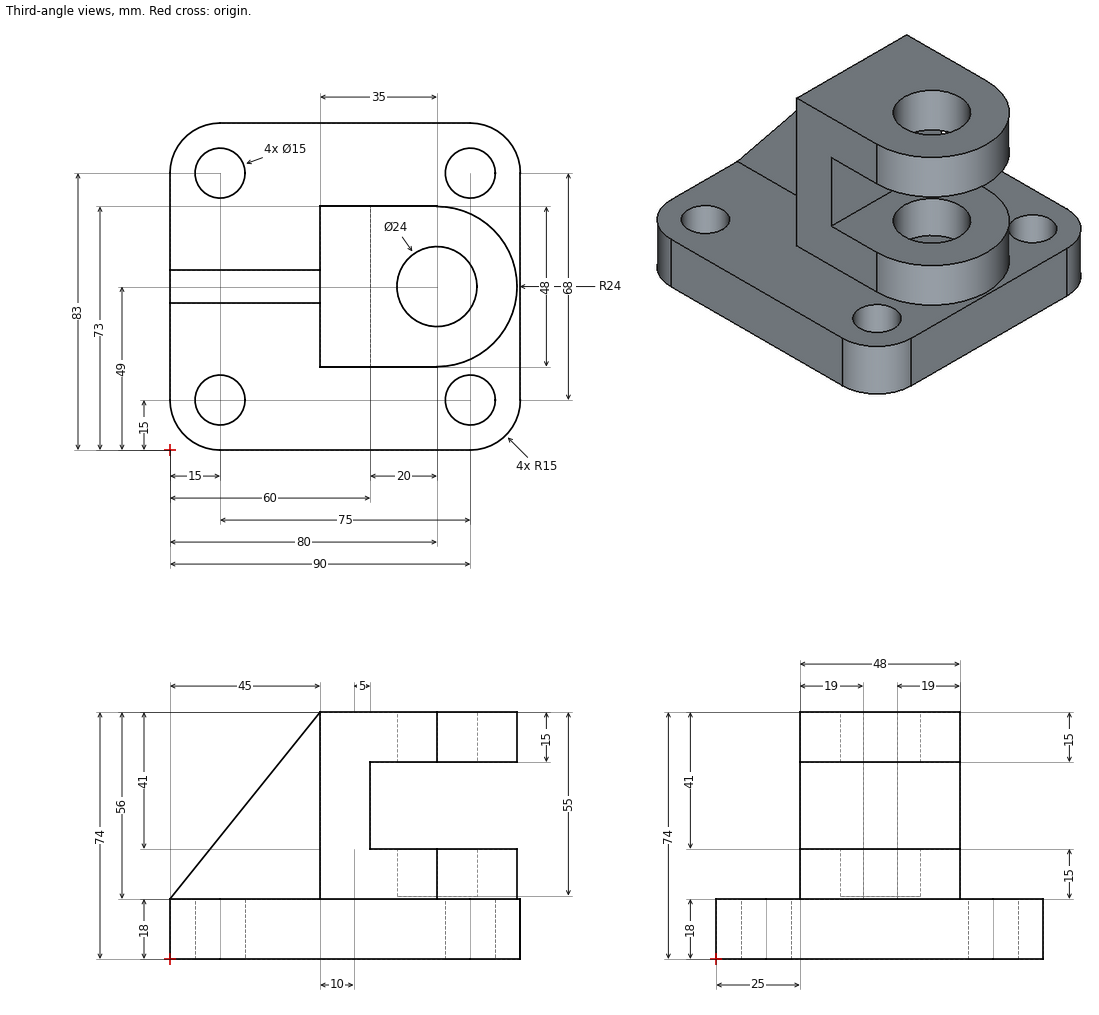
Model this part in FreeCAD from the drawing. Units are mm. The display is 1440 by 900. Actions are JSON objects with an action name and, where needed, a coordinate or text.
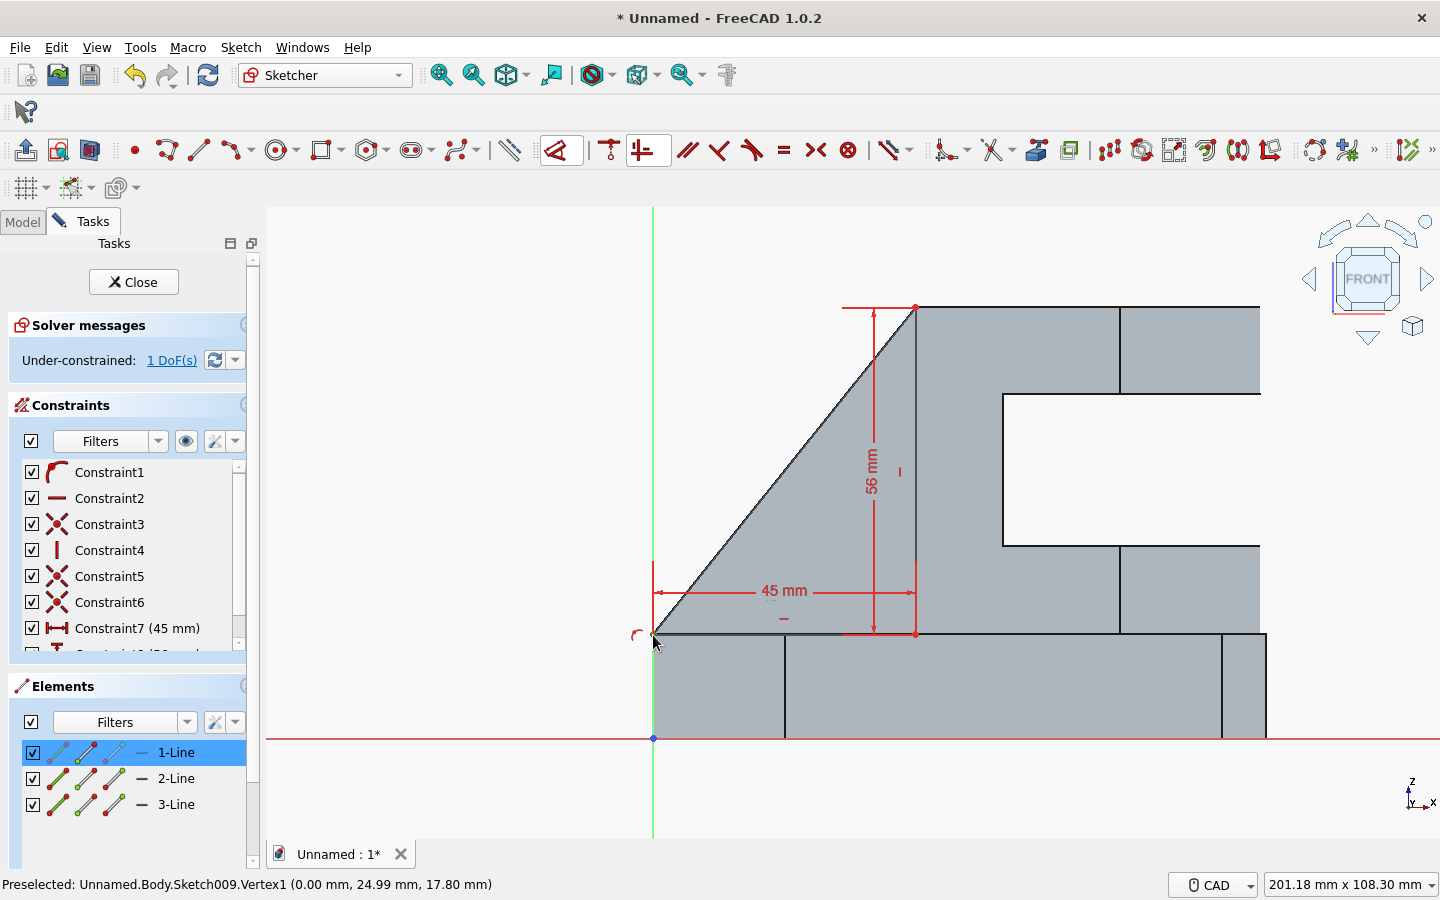
{"action": "left_click", "coordinate": [578, 150]}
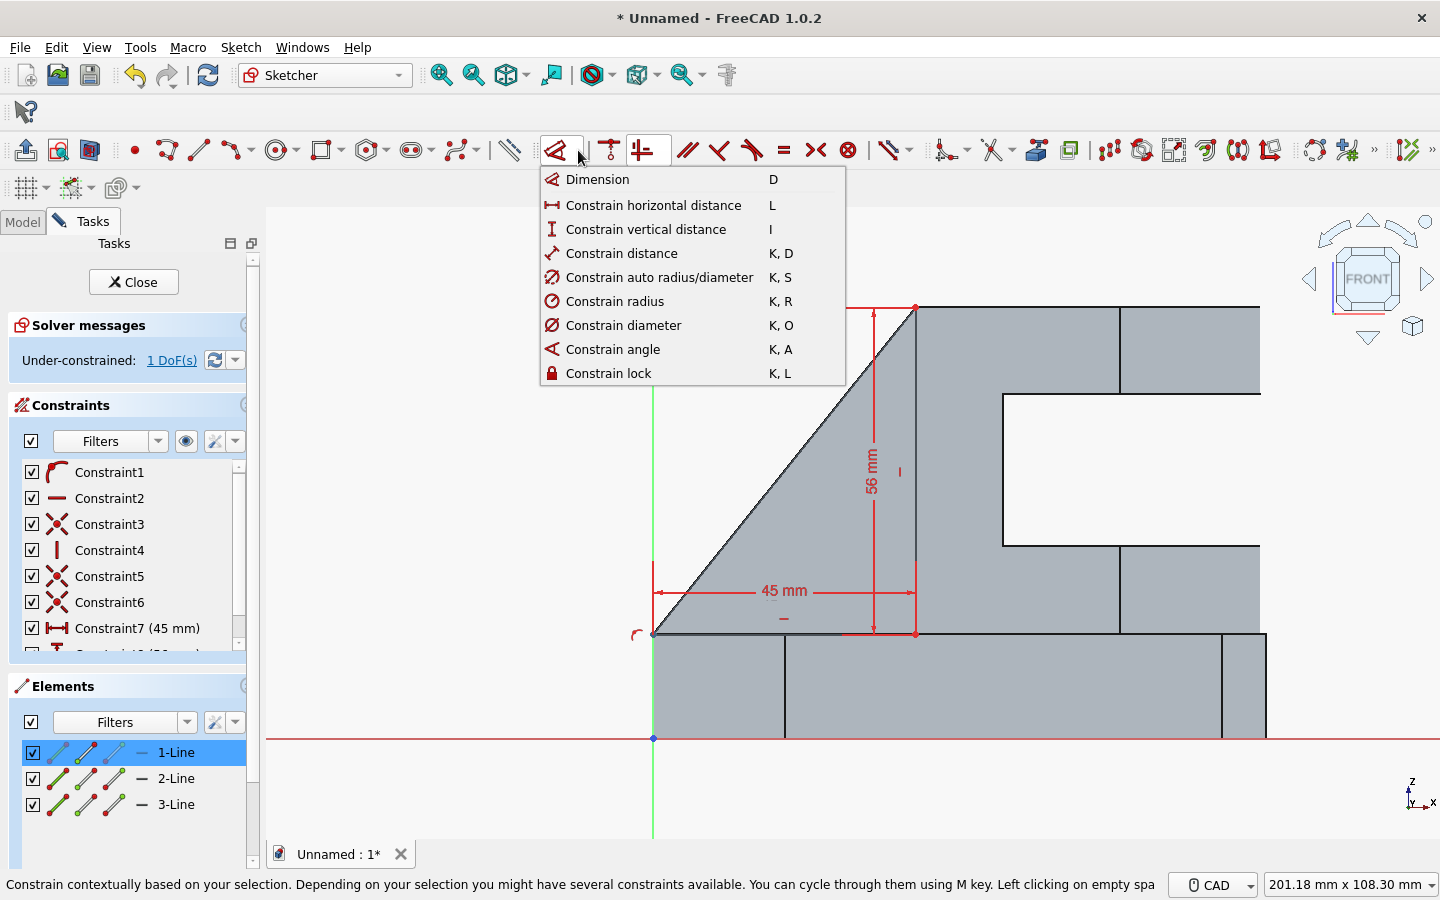
{"action": "left_click", "coordinate": [693, 229]}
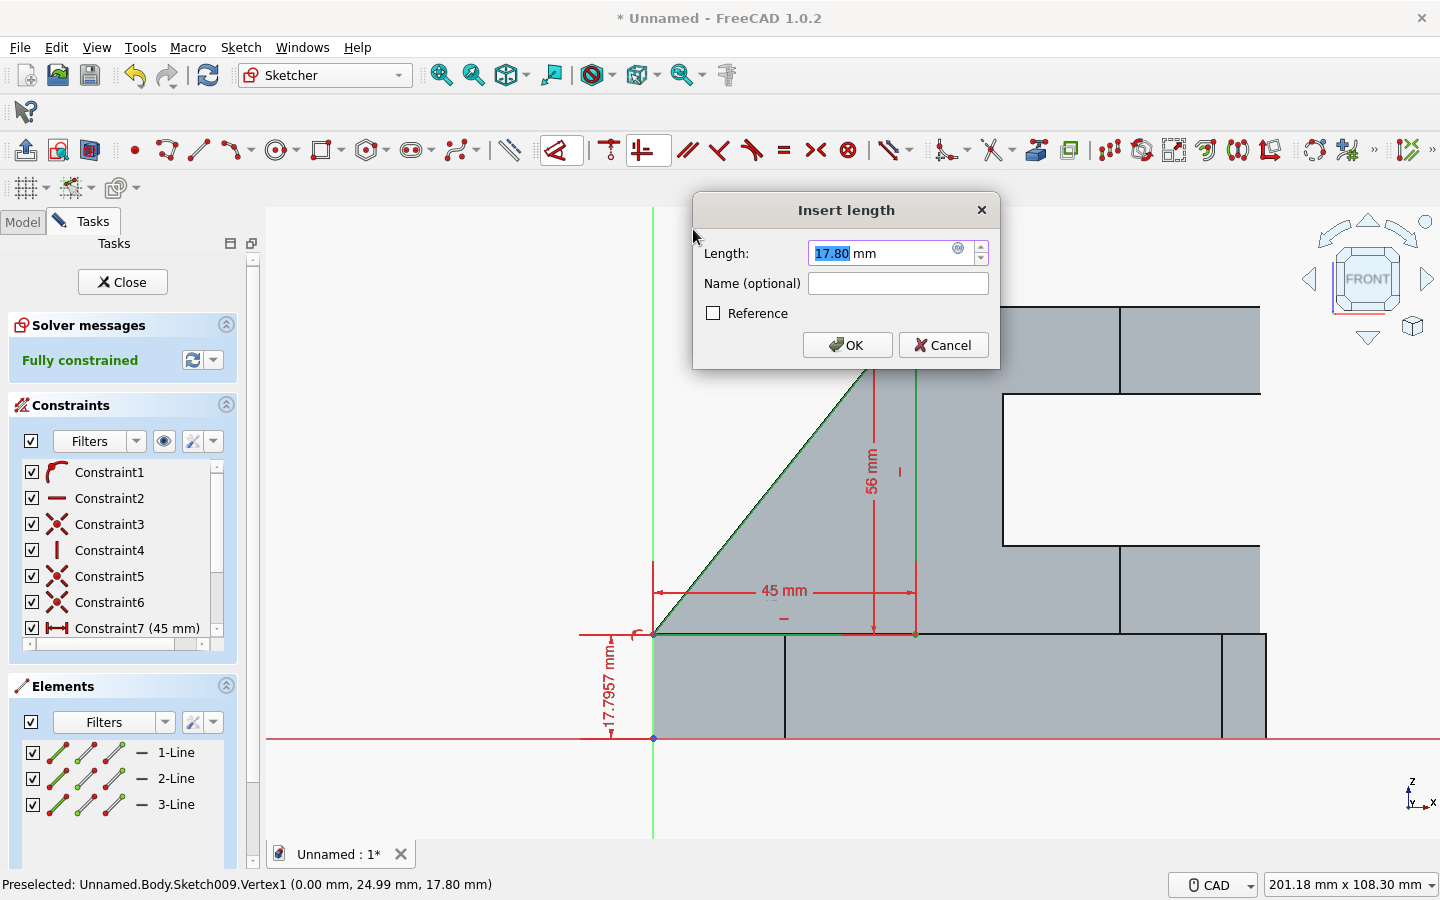
{"action": "type", "text": "18"}
{"action": "key", "text": "Return"}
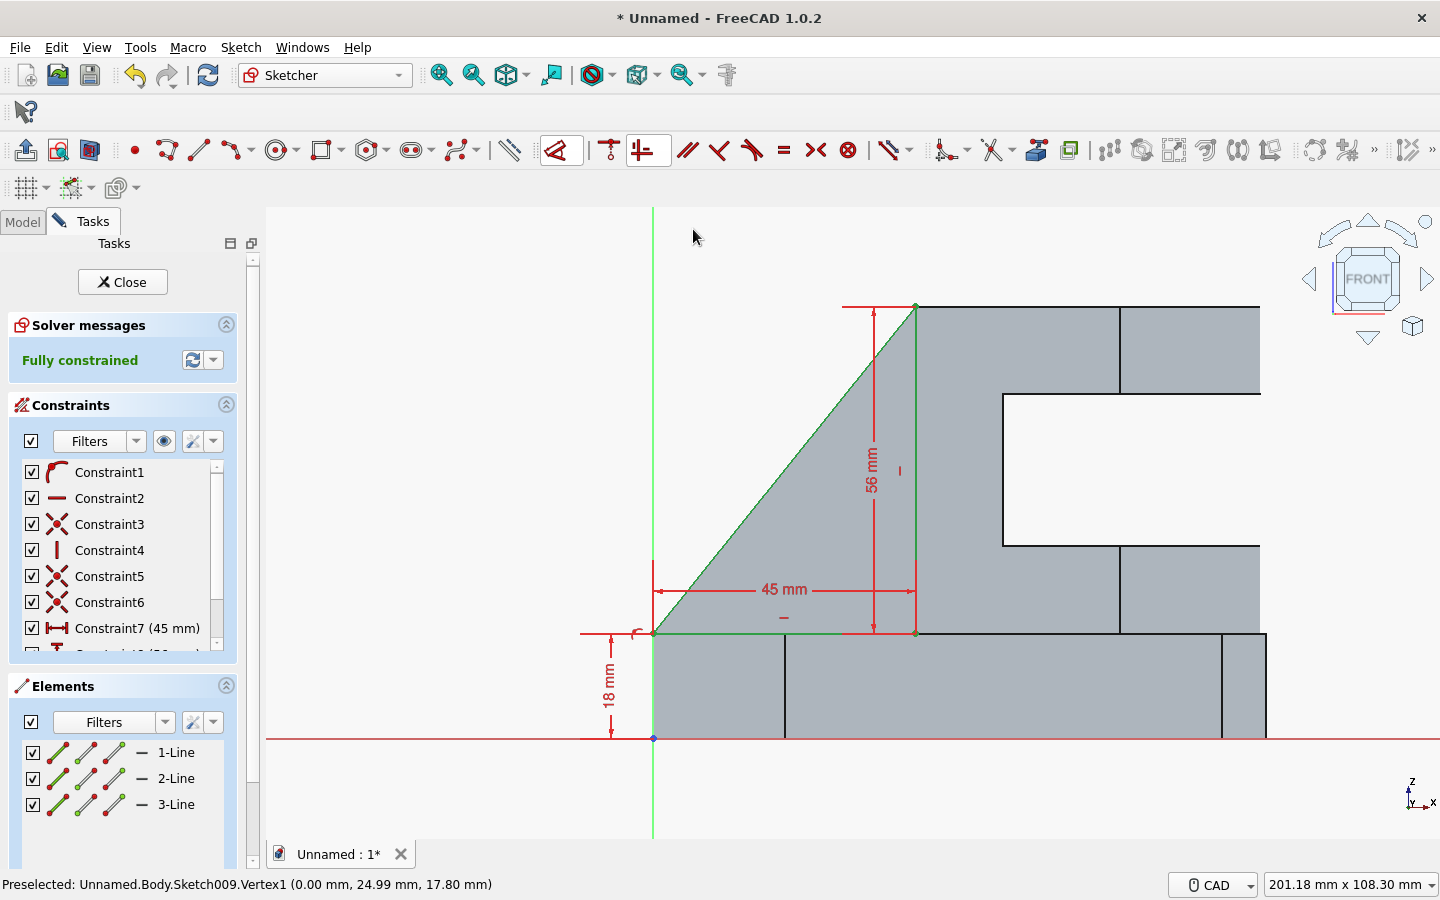
{"action": "left_click", "coordinate": [123, 282]}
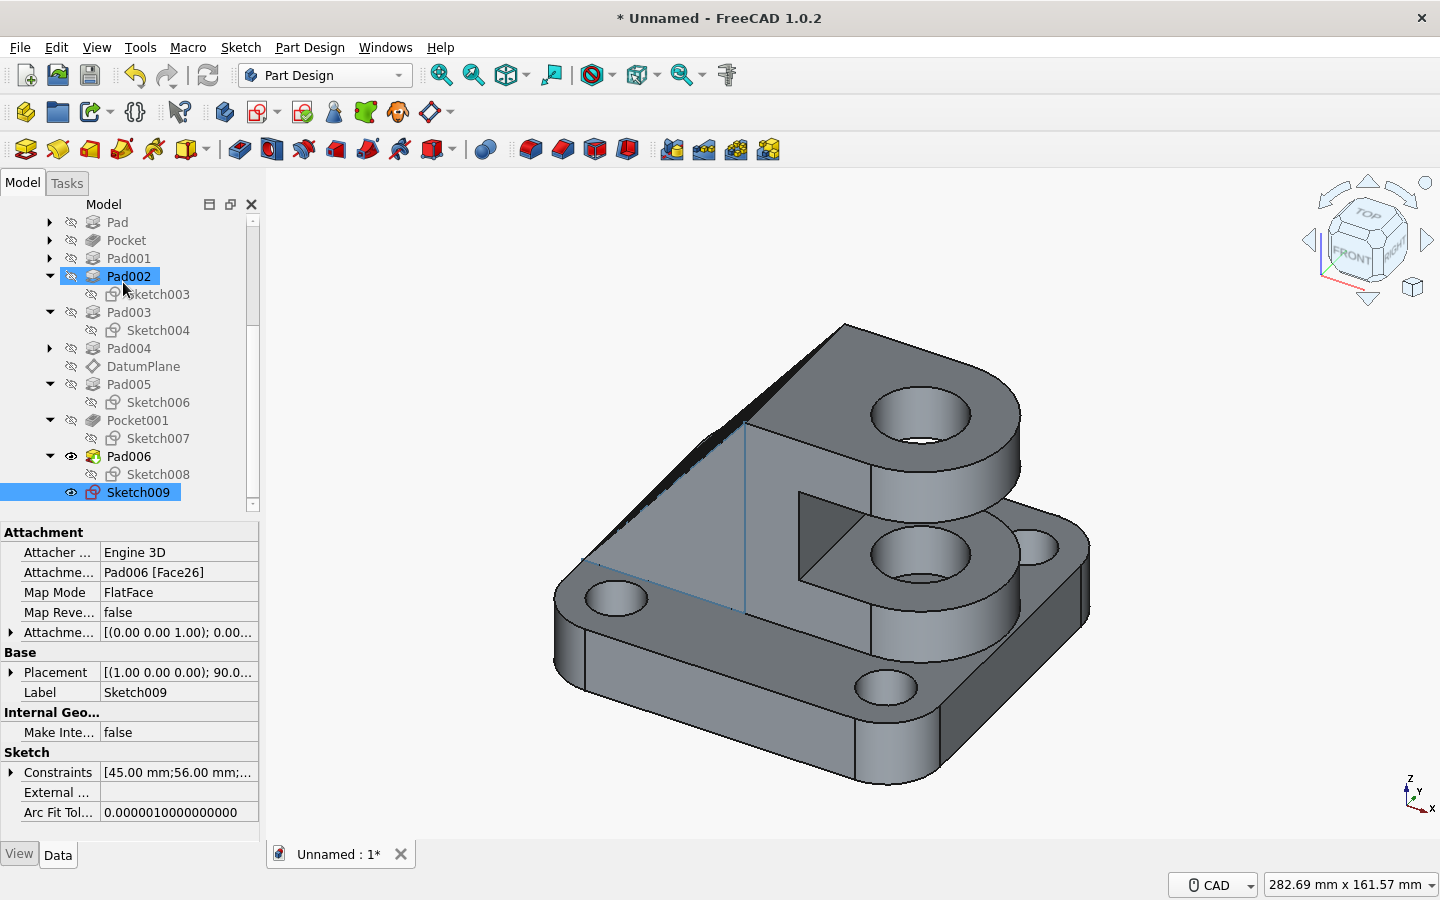
{"action": "left_click", "coordinate": [240, 150]}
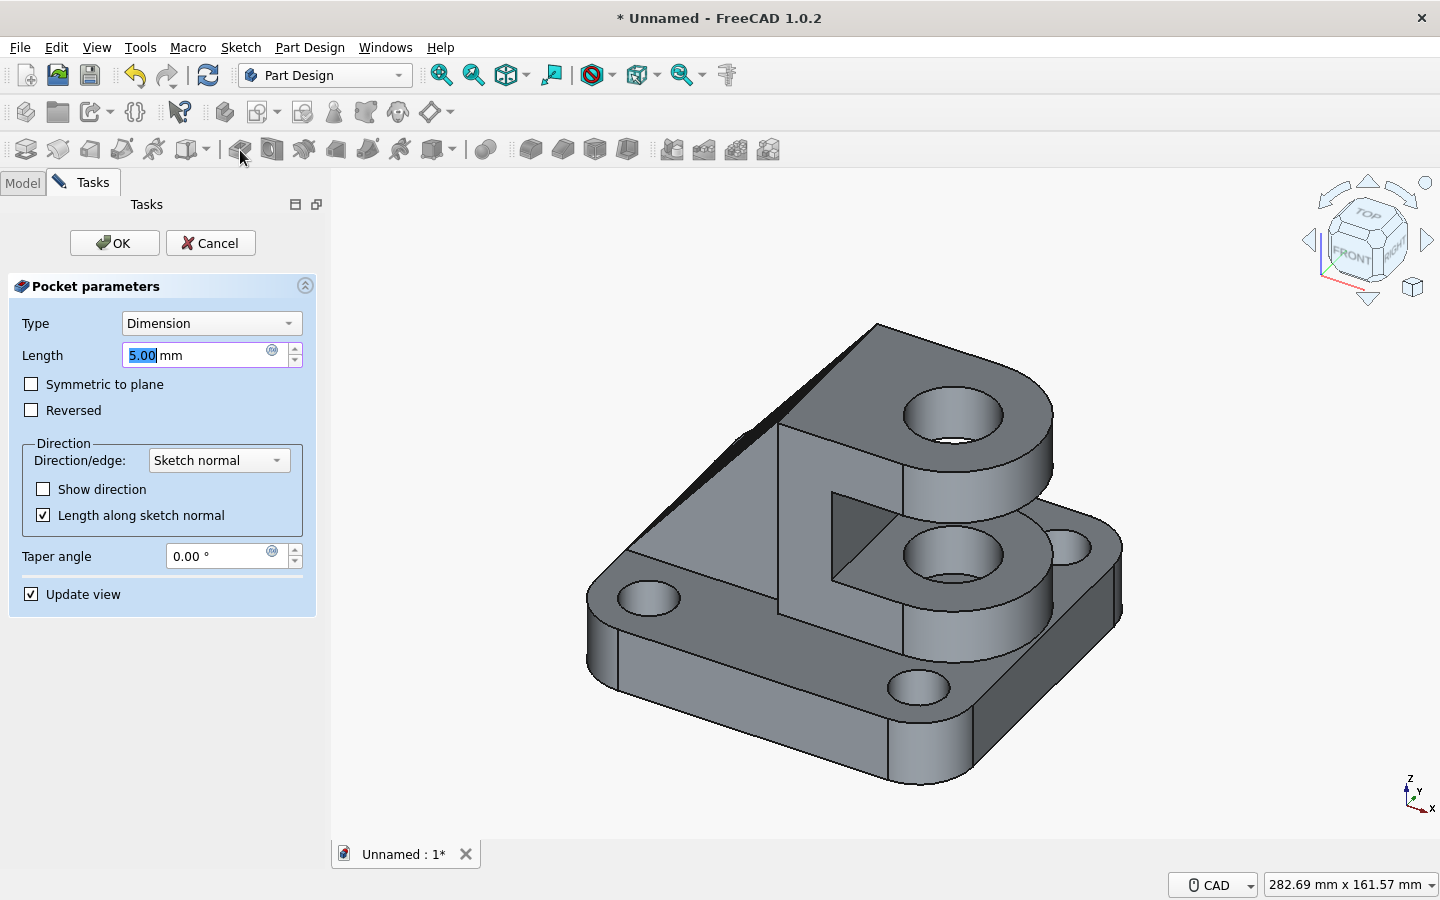
{"action": "type", "text": "19"}
{"action": "key", "text": "Tab"}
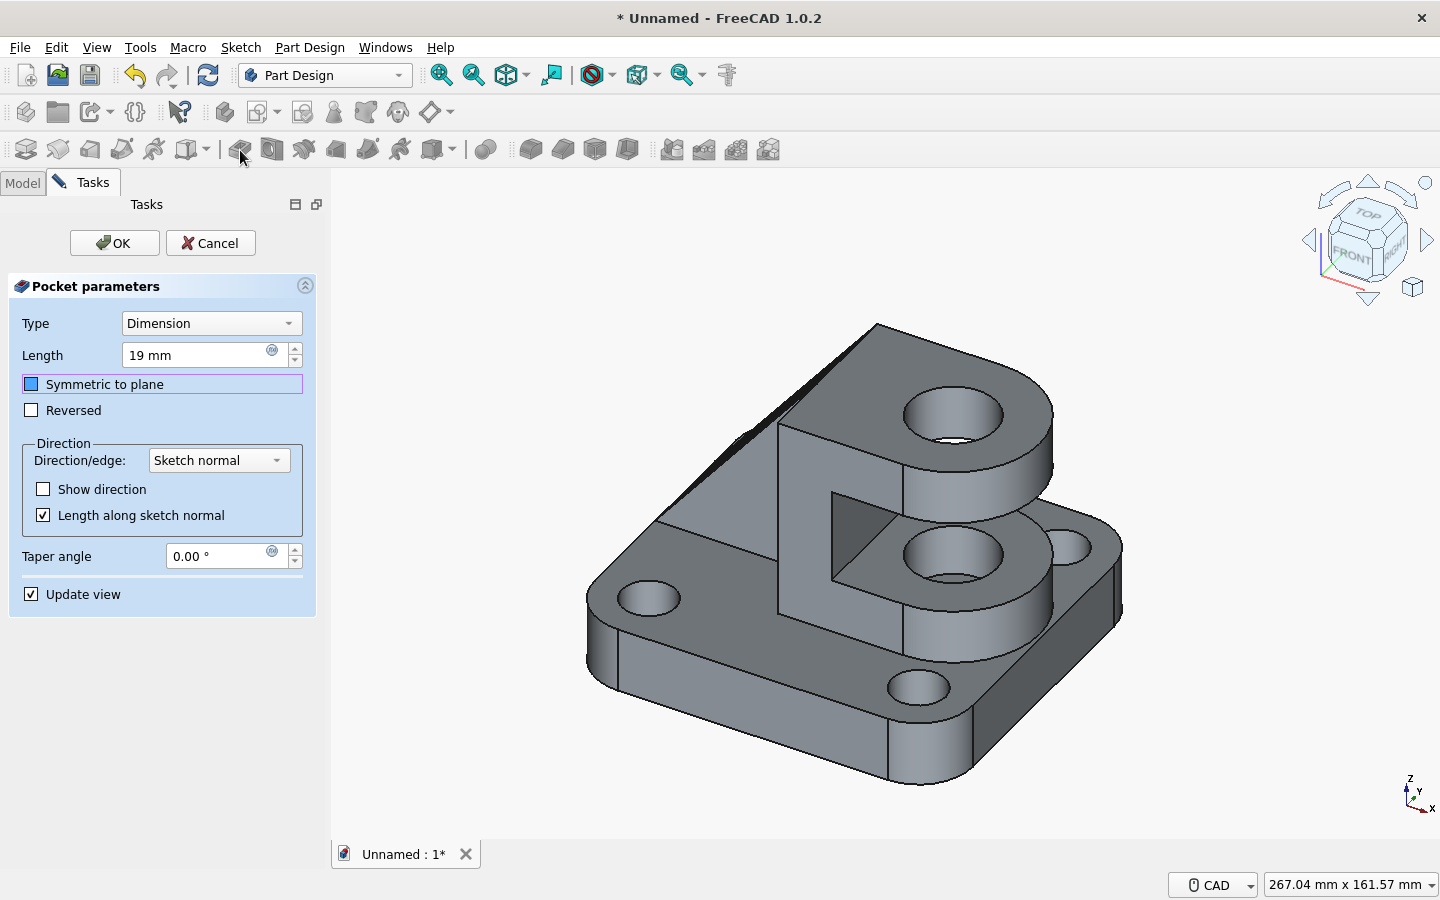
{"action": "left_click", "coordinate": [115, 243]}